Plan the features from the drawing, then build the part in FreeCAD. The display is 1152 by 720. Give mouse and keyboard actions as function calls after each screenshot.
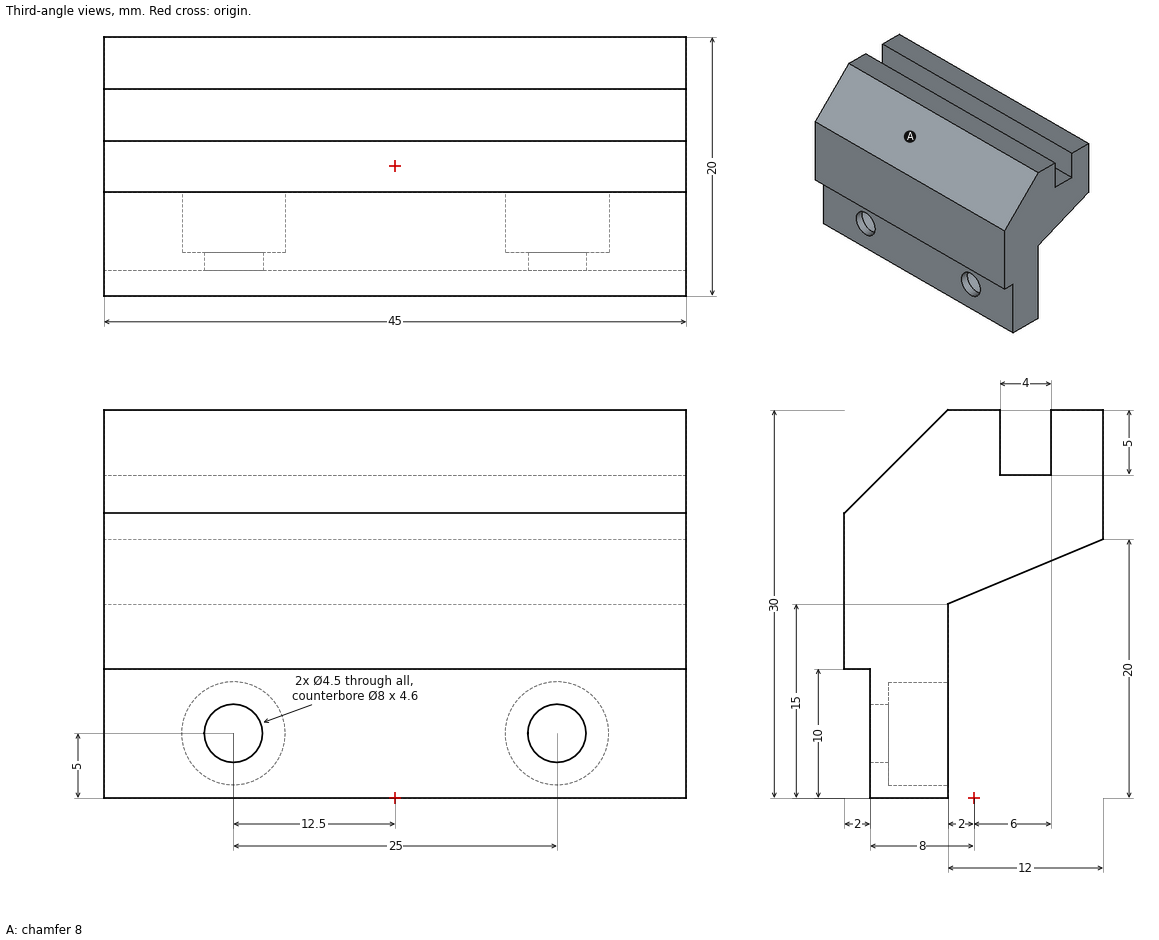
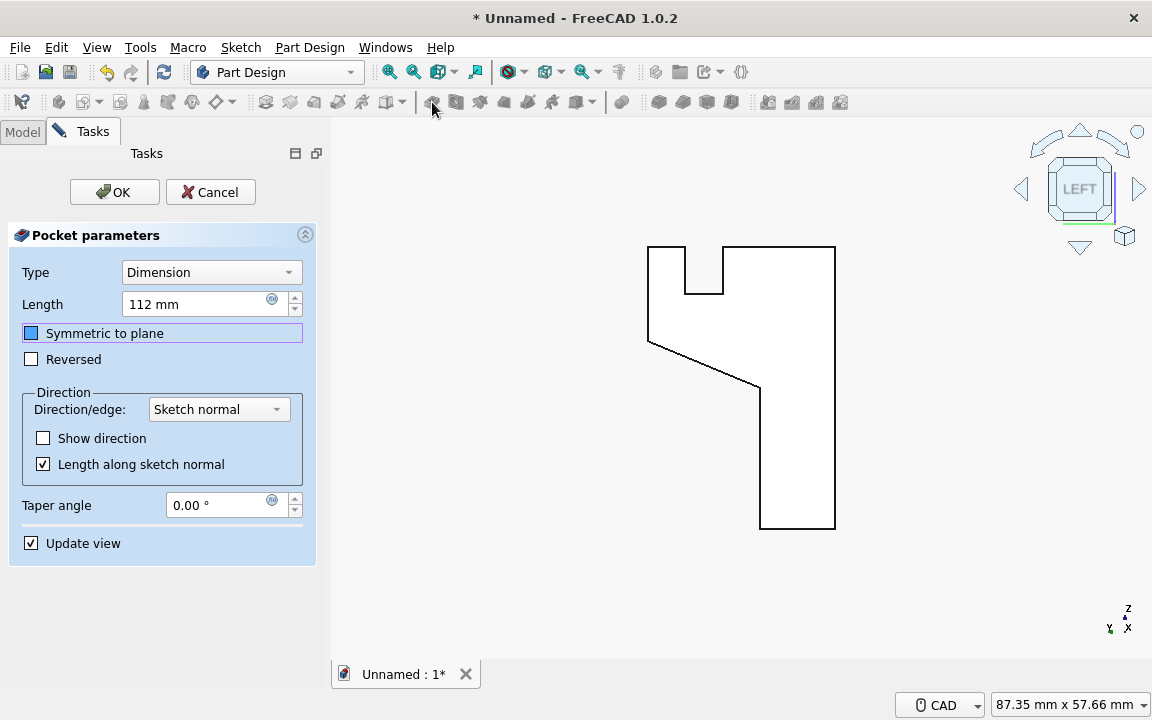
click(30, 333)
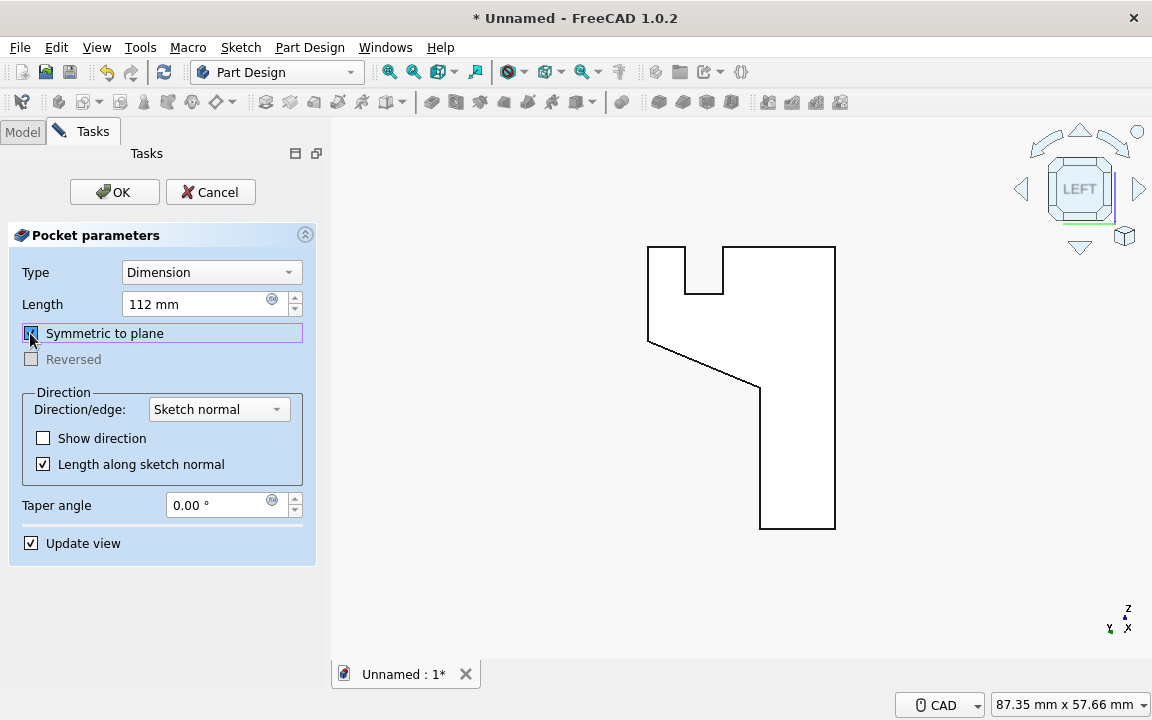
click(115, 192)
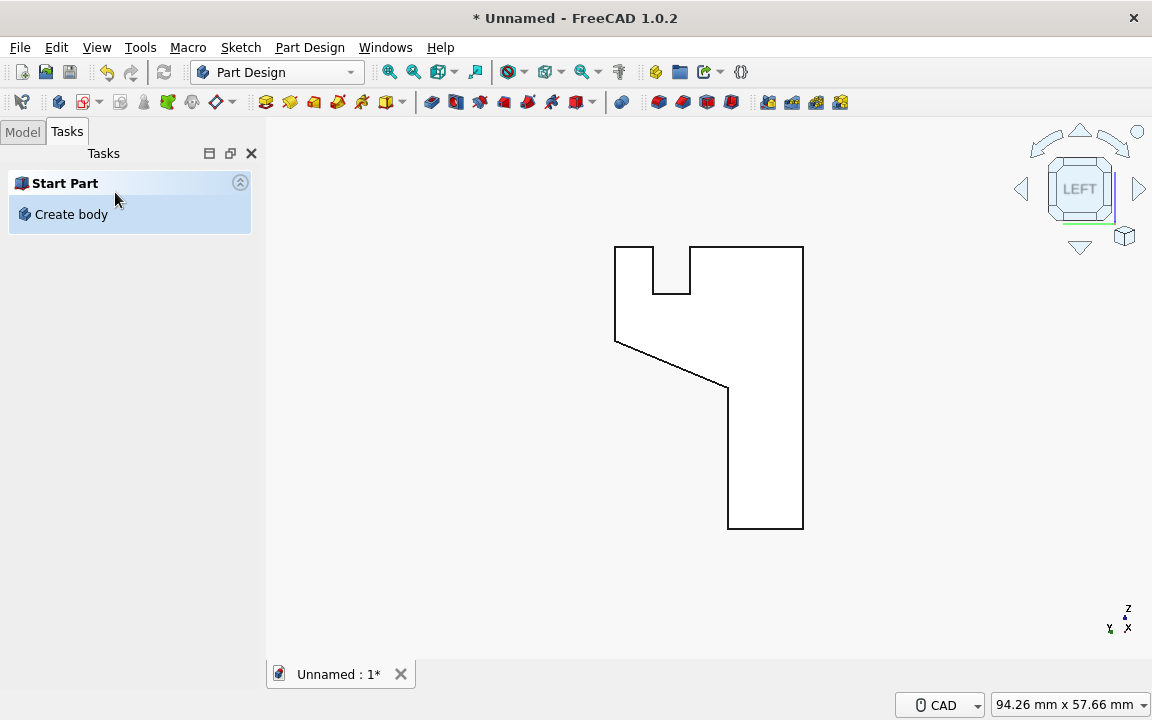
key(0)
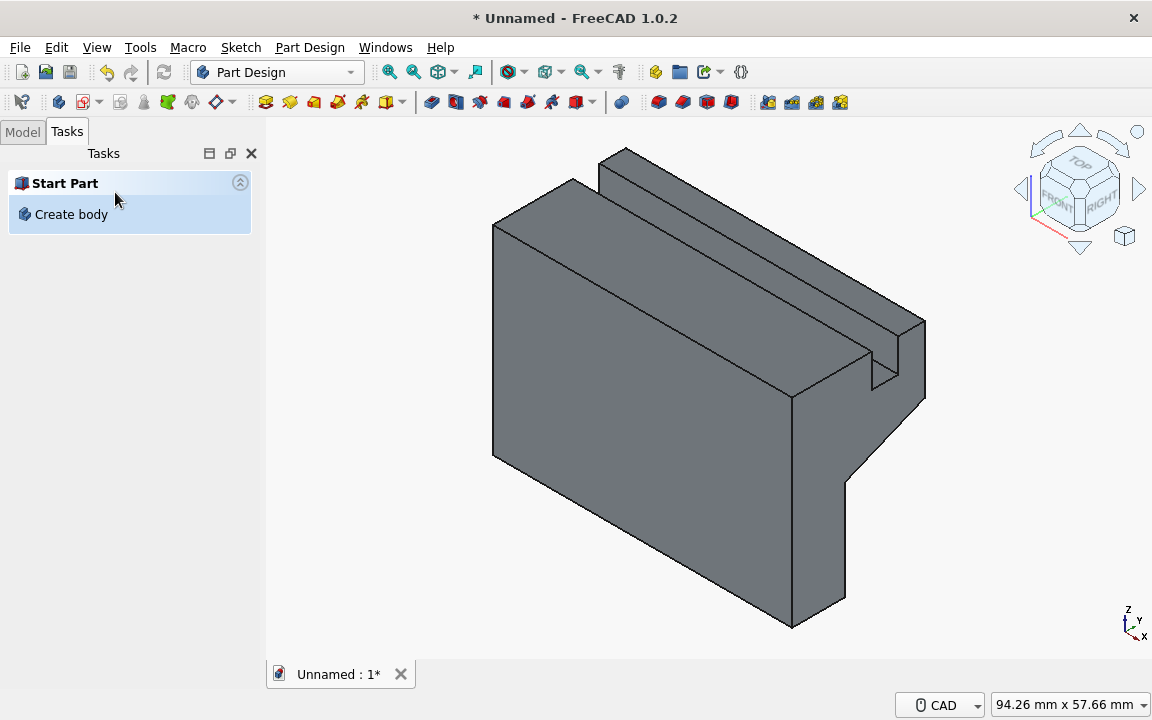
click(643, 310)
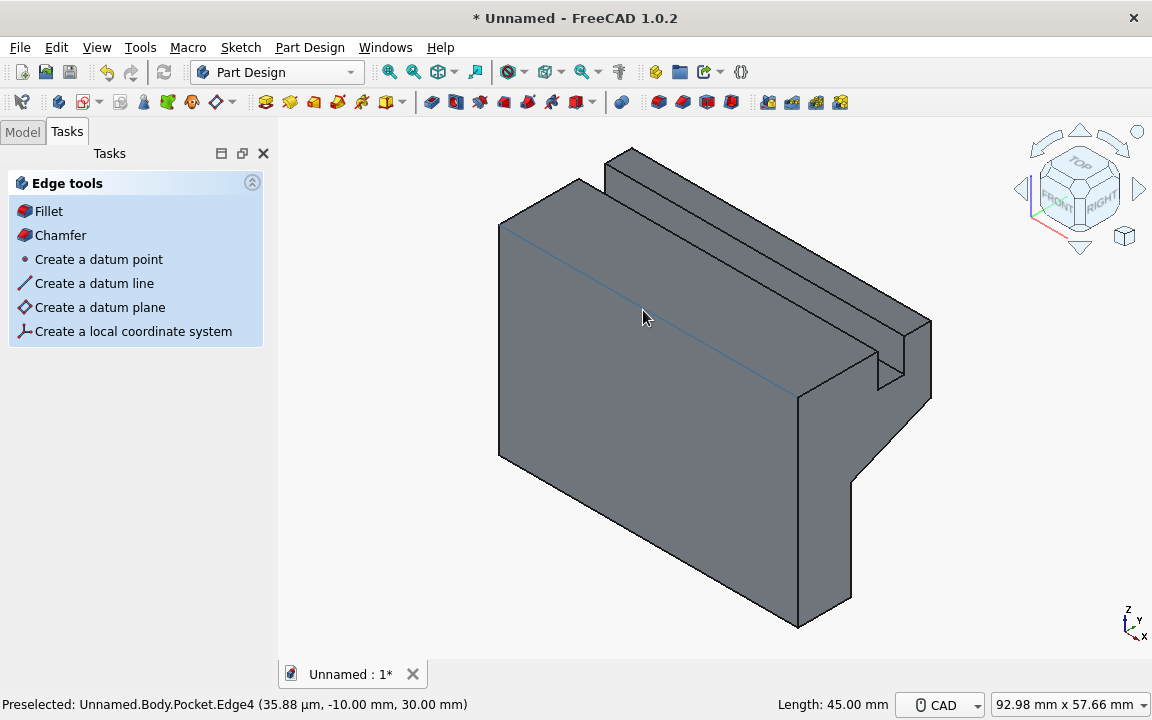
click(684, 102)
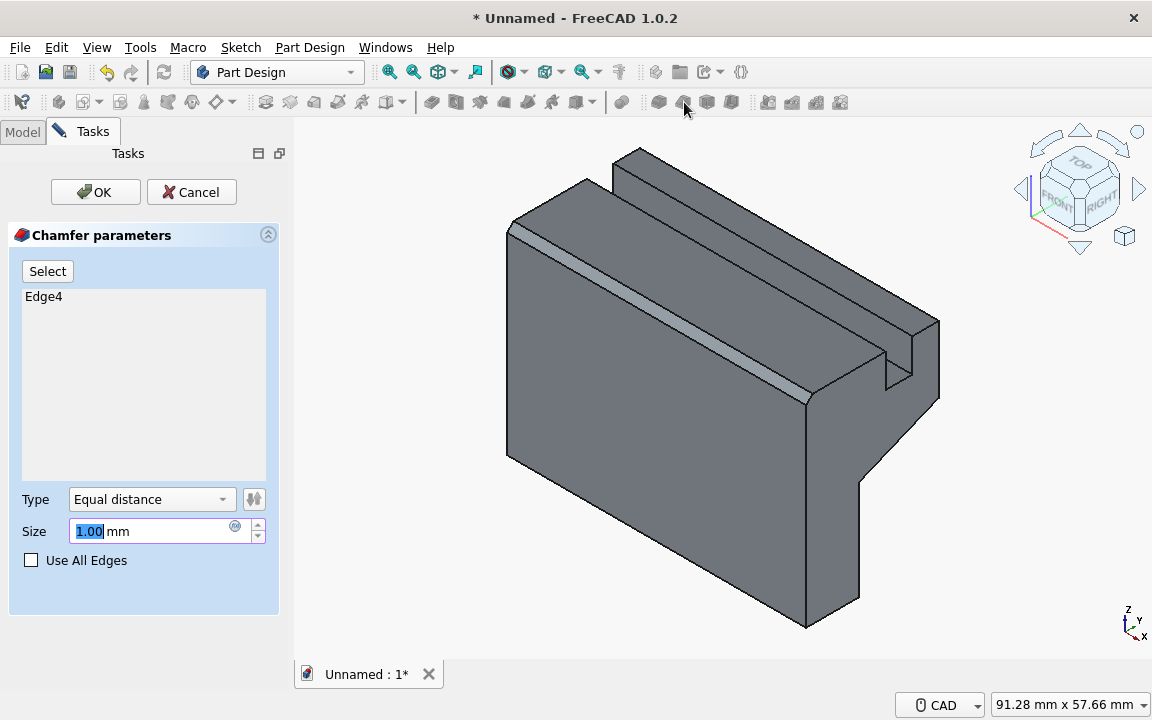
text(8)
key(Tab)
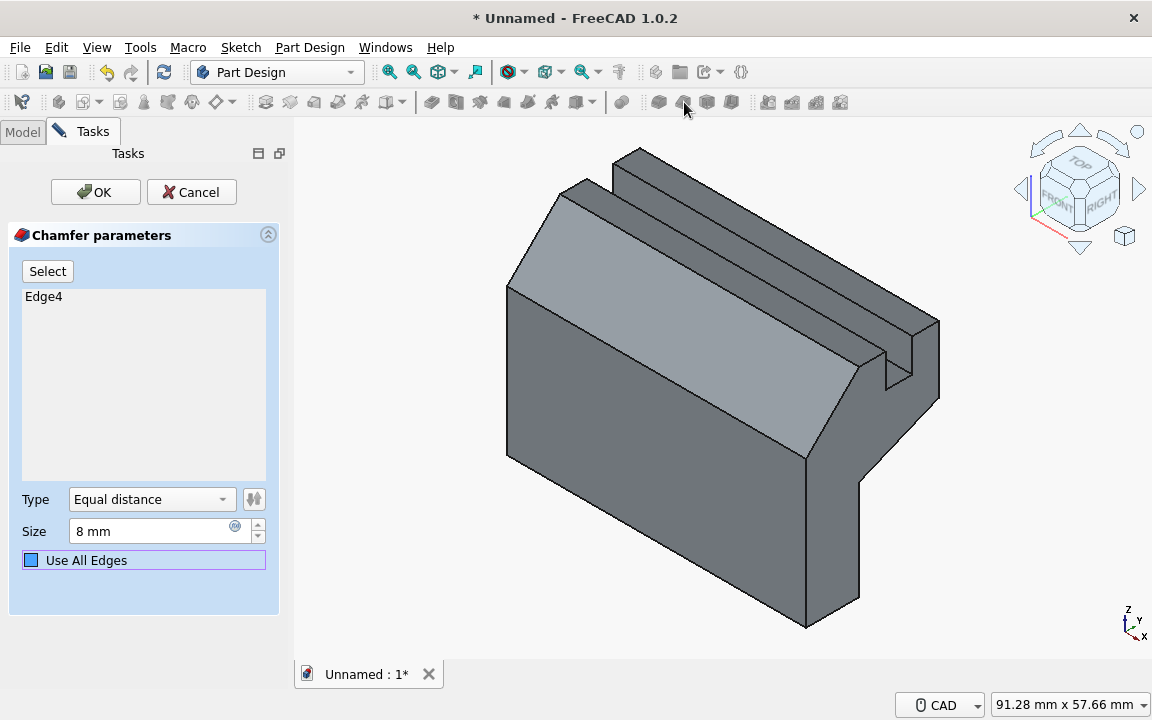
click(96, 192)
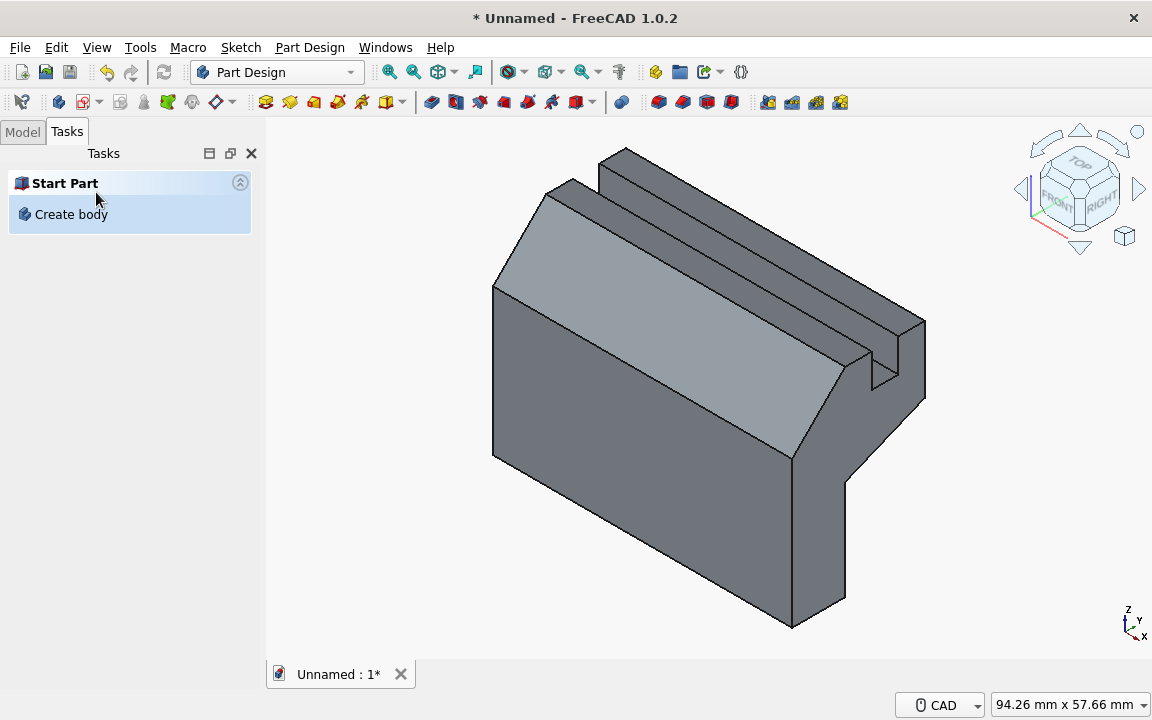
key(4)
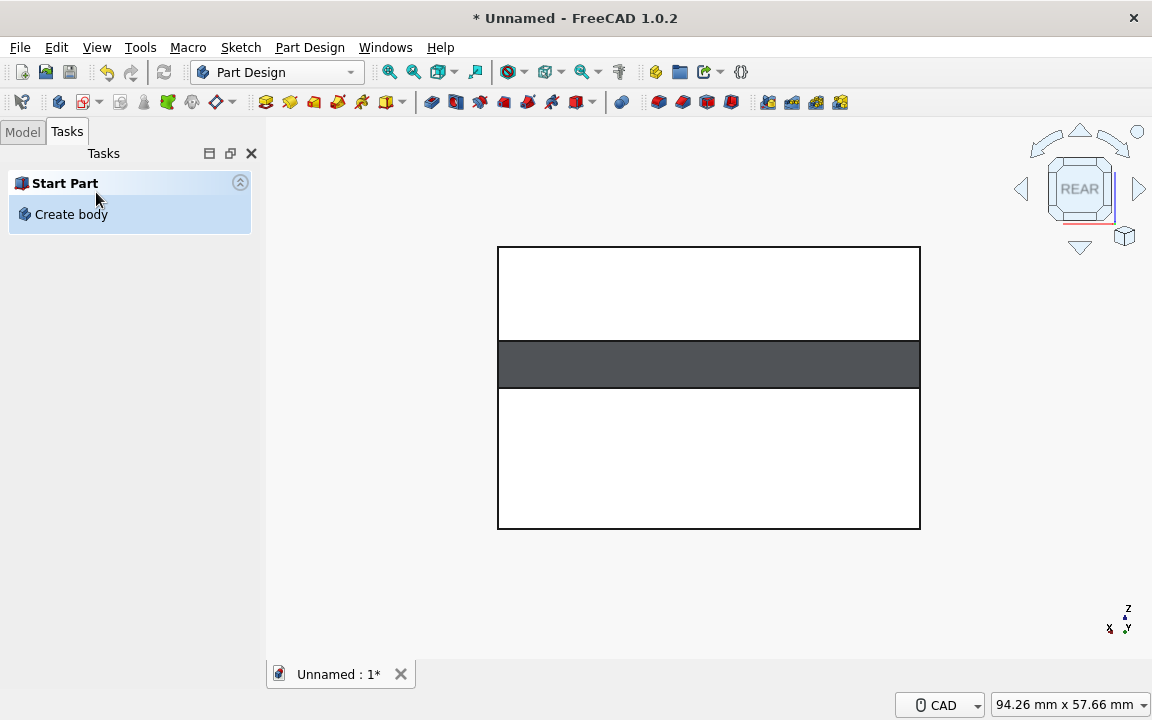
click(588, 457)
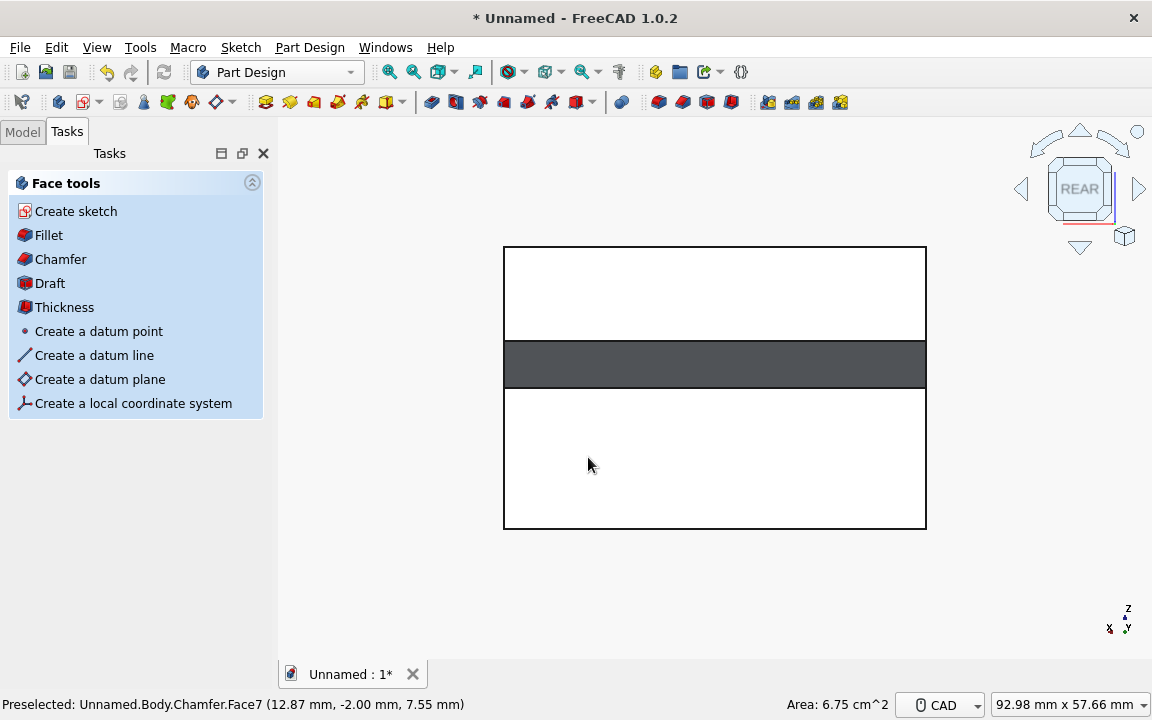
click(84, 102)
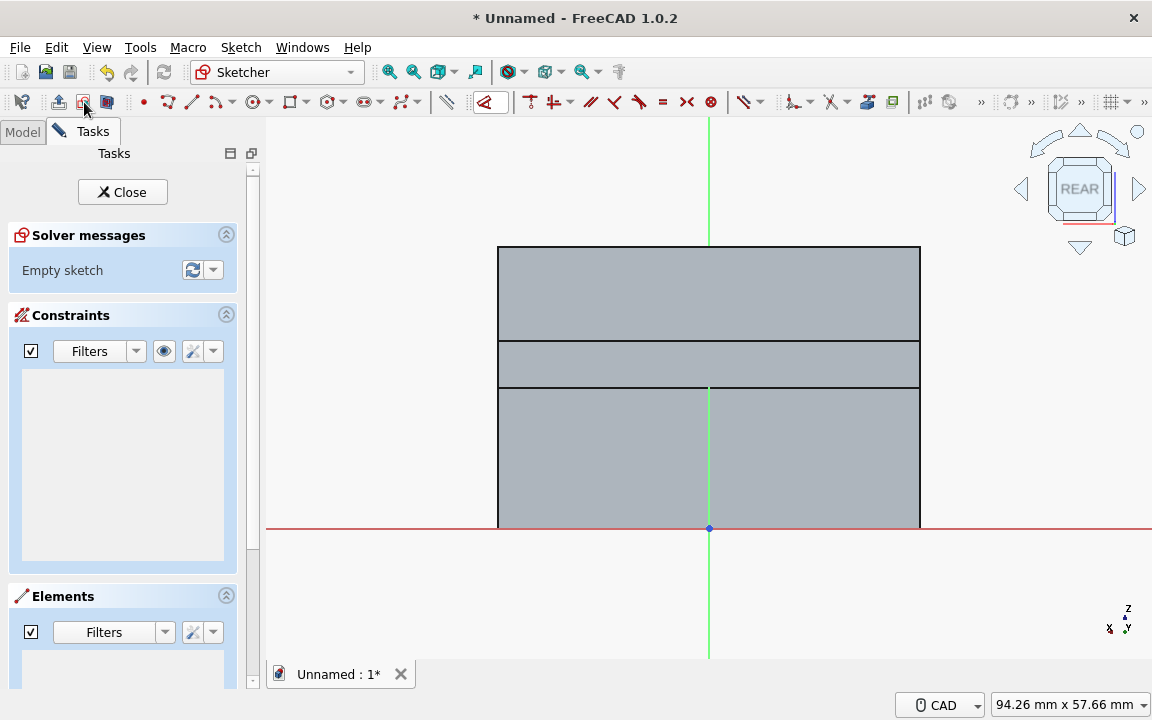
key(q)
key(s)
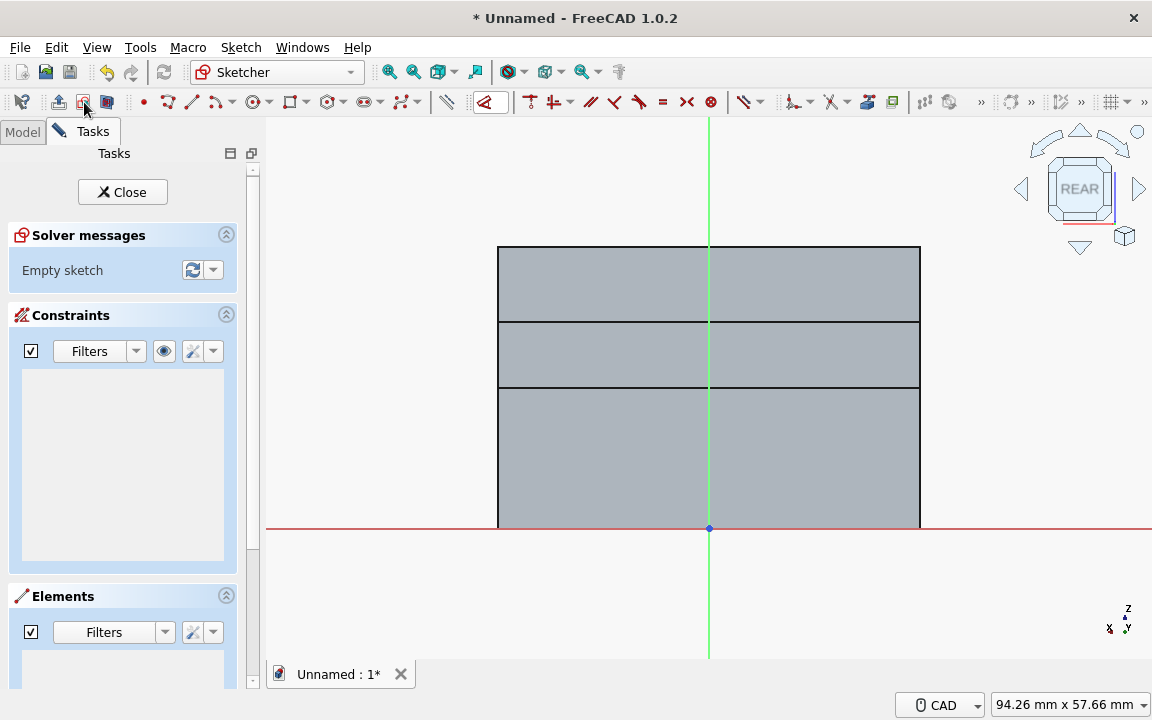
scroll(792, 625, up, 3)